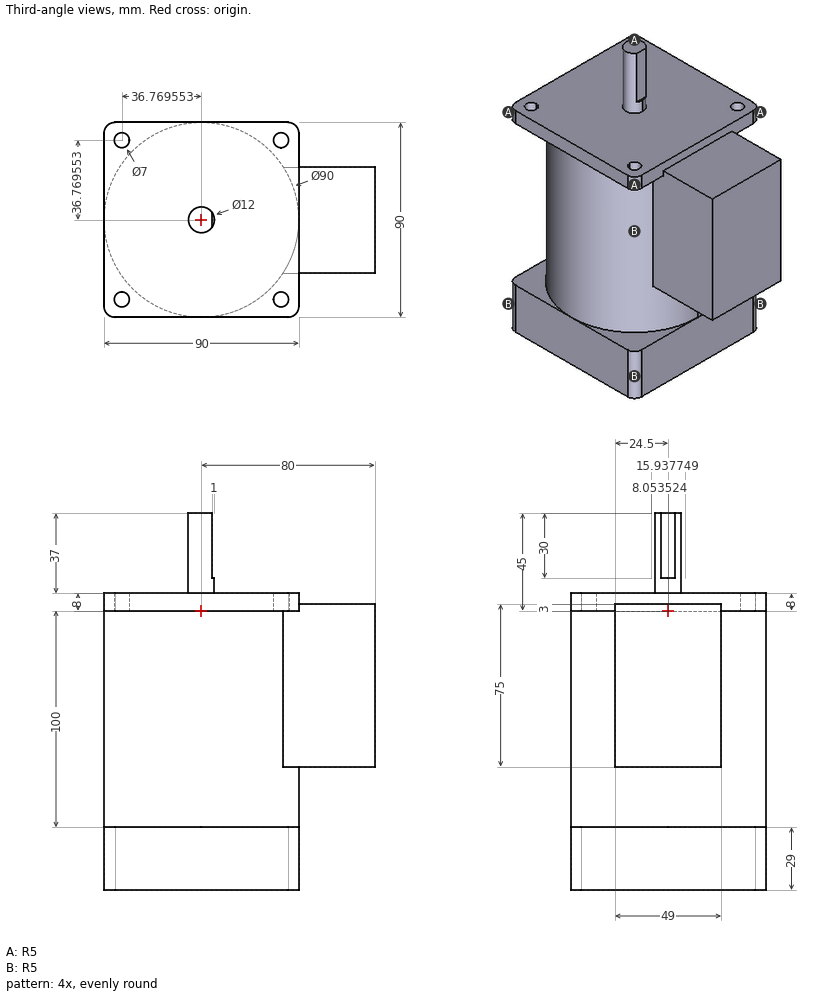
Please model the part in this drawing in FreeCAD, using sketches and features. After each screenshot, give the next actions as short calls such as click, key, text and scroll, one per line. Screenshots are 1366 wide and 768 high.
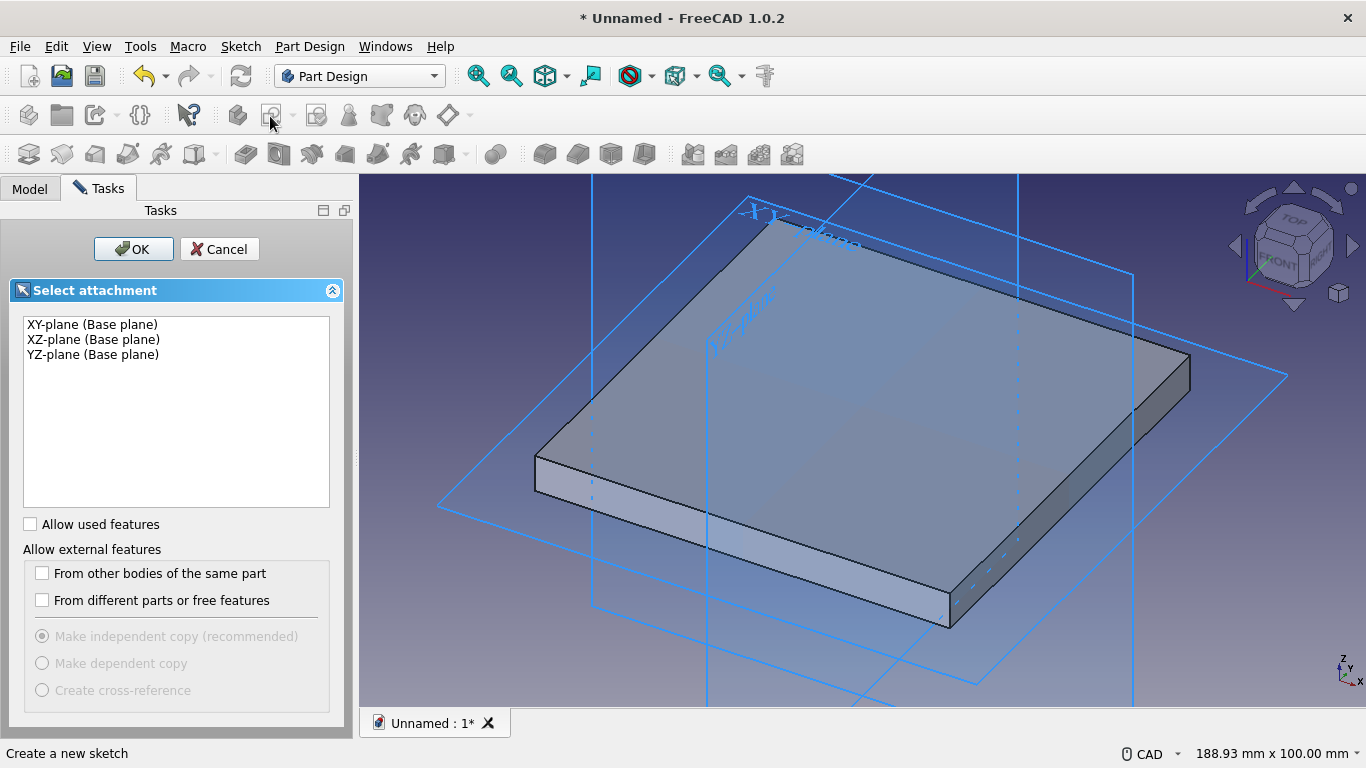
click(84, 324)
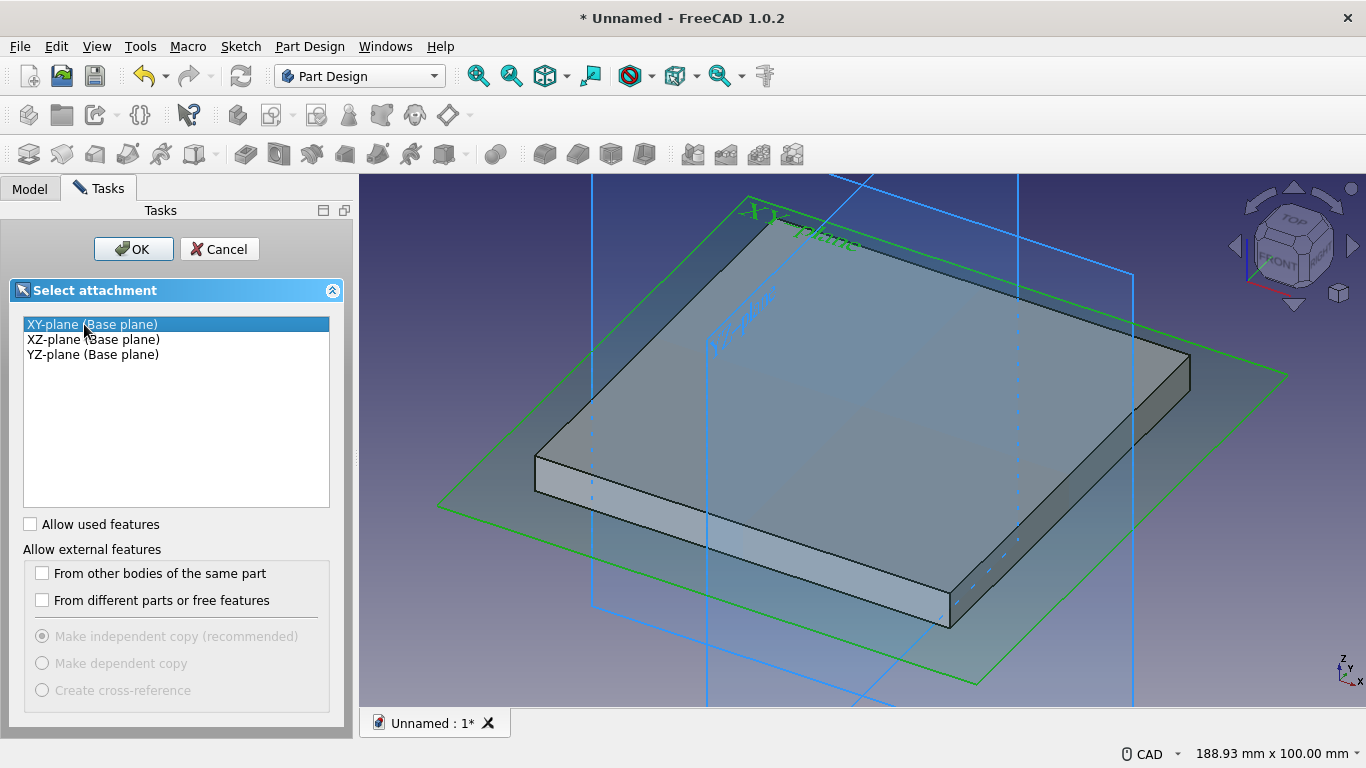
click(134, 249)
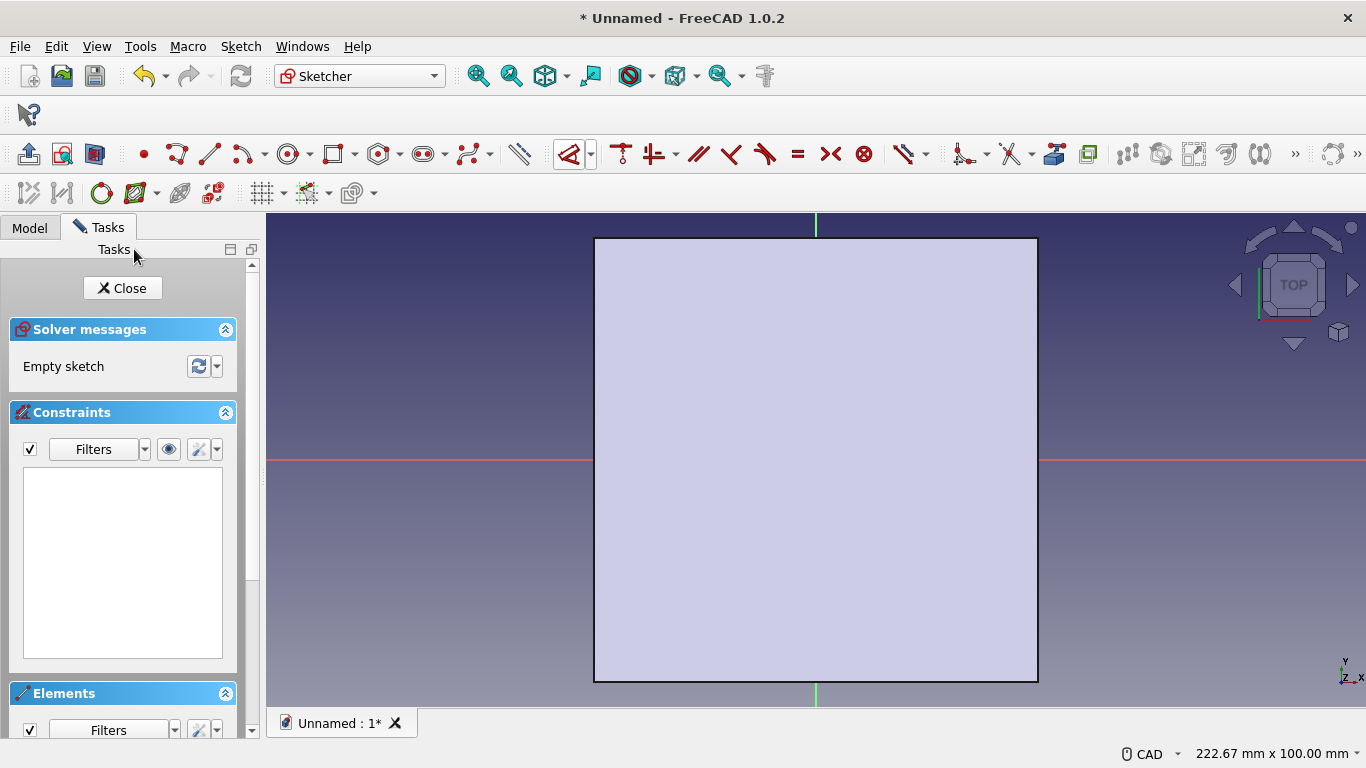
click(95, 154)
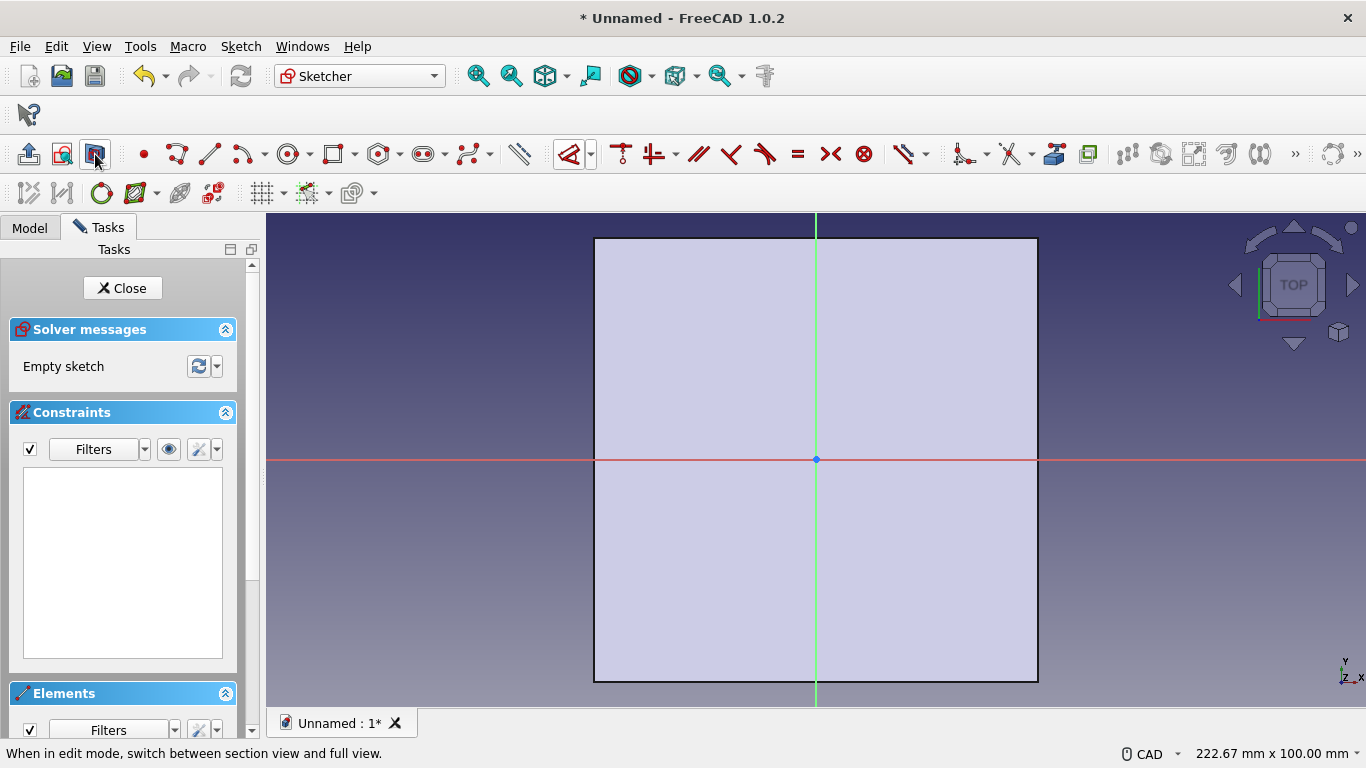
scroll(608, 460, down, 2)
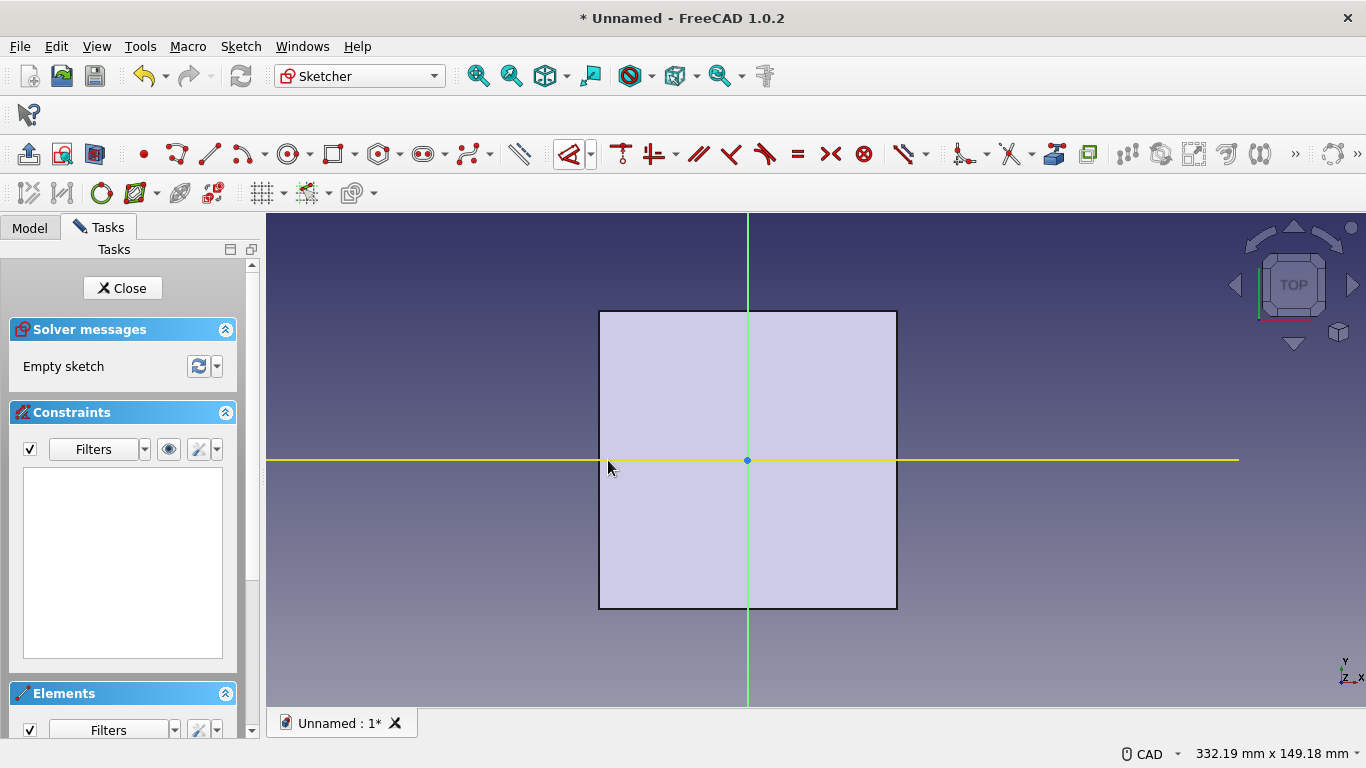
key(g)
key(c)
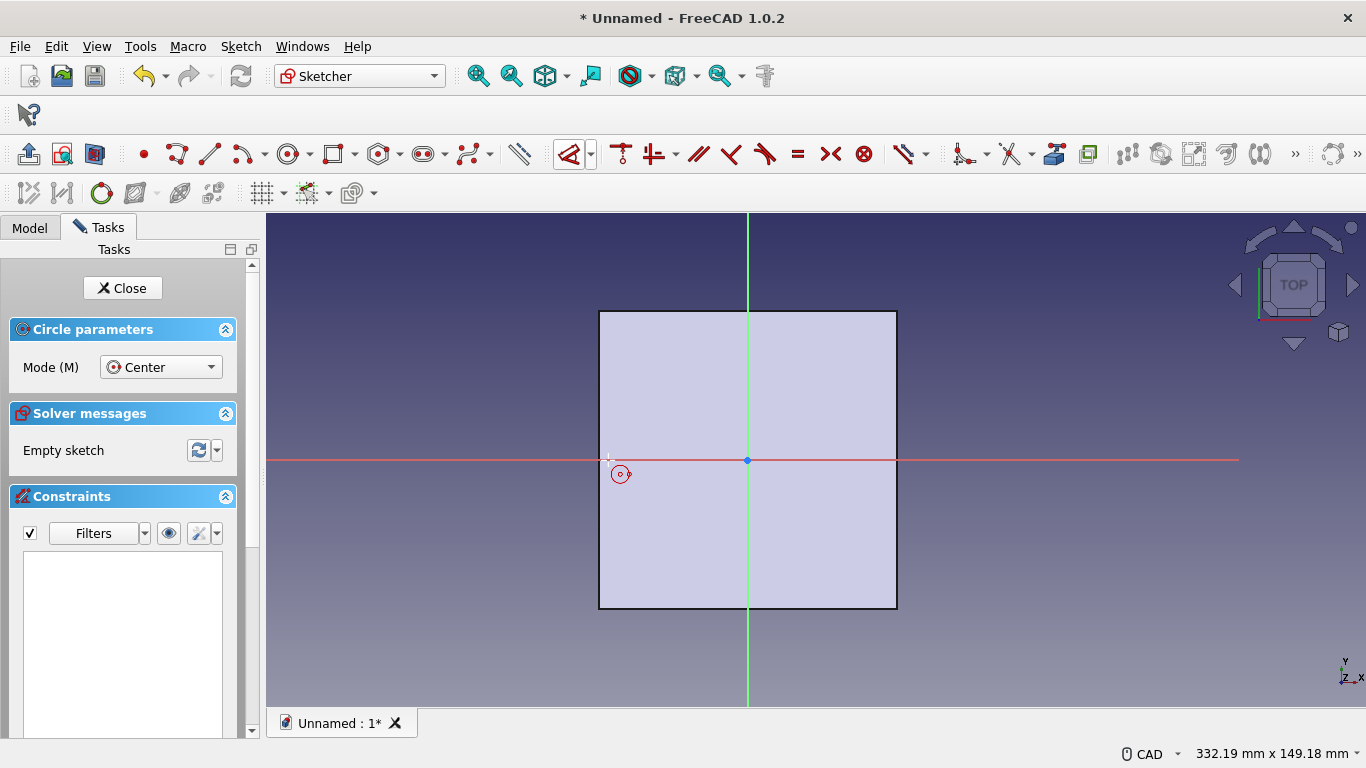
click(748, 460)
click(853, 355)
key(Escape)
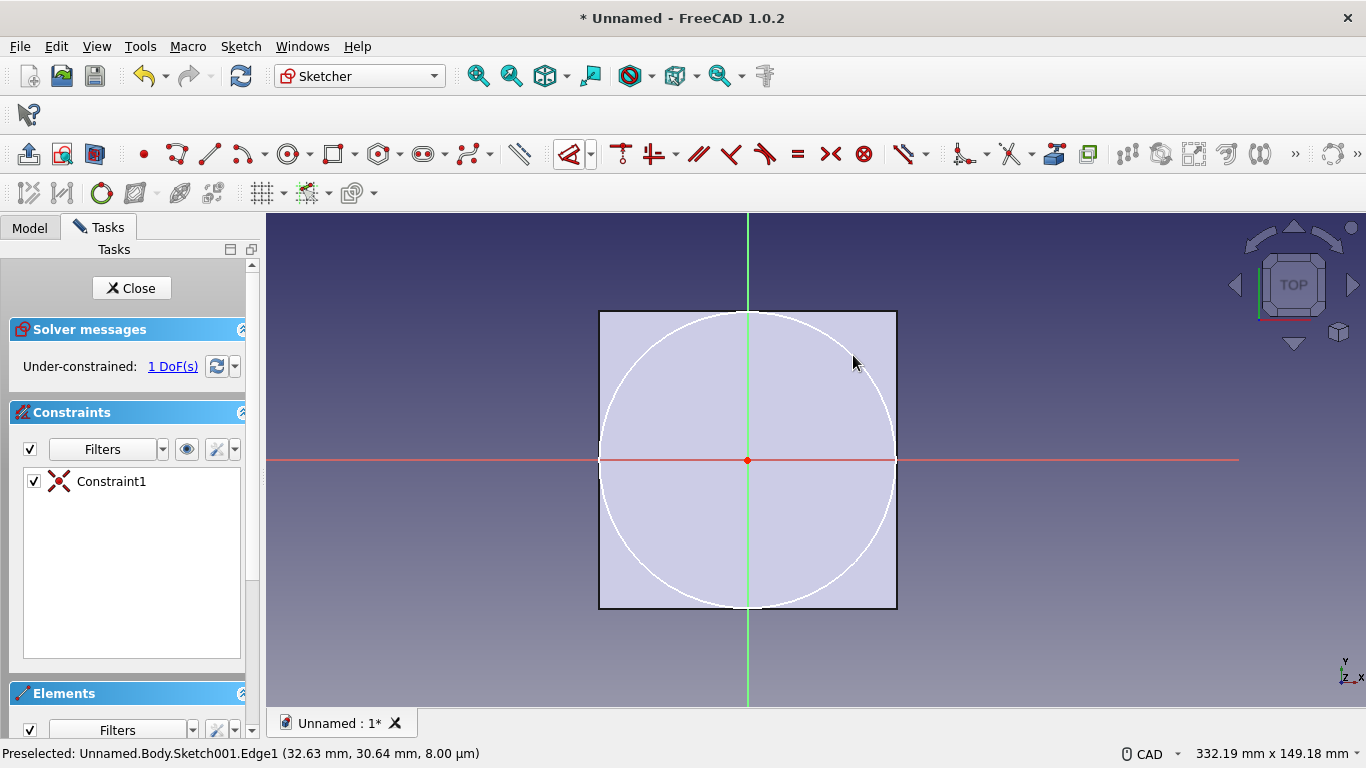
click(852, 355)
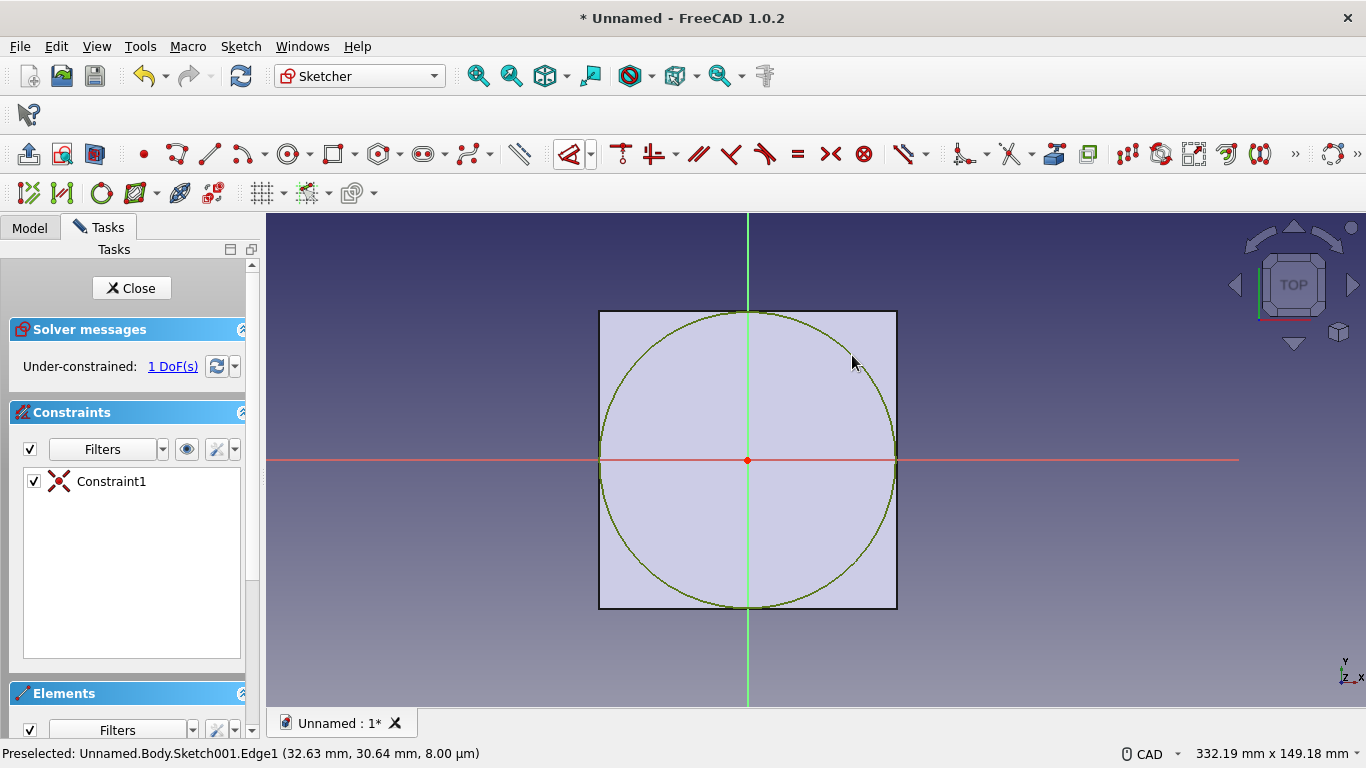
click(590, 154)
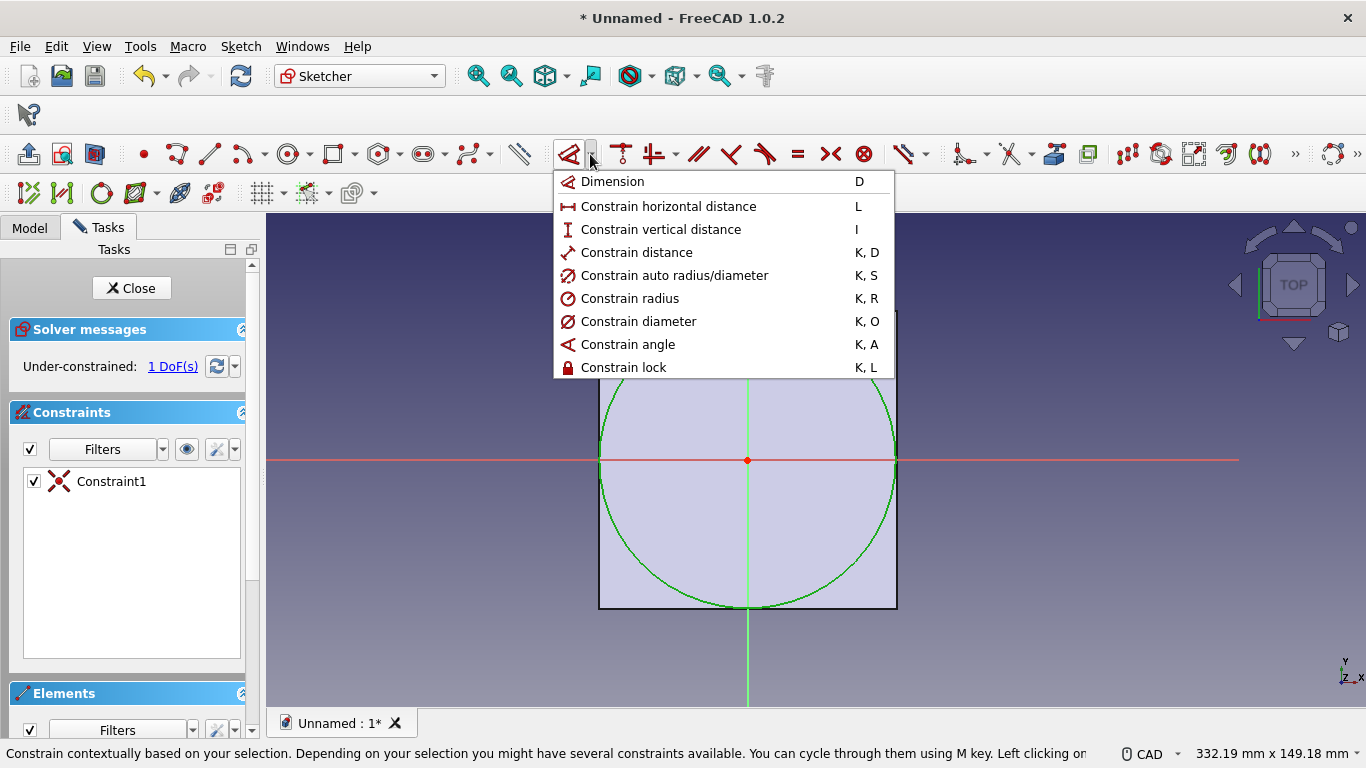
click(724, 322)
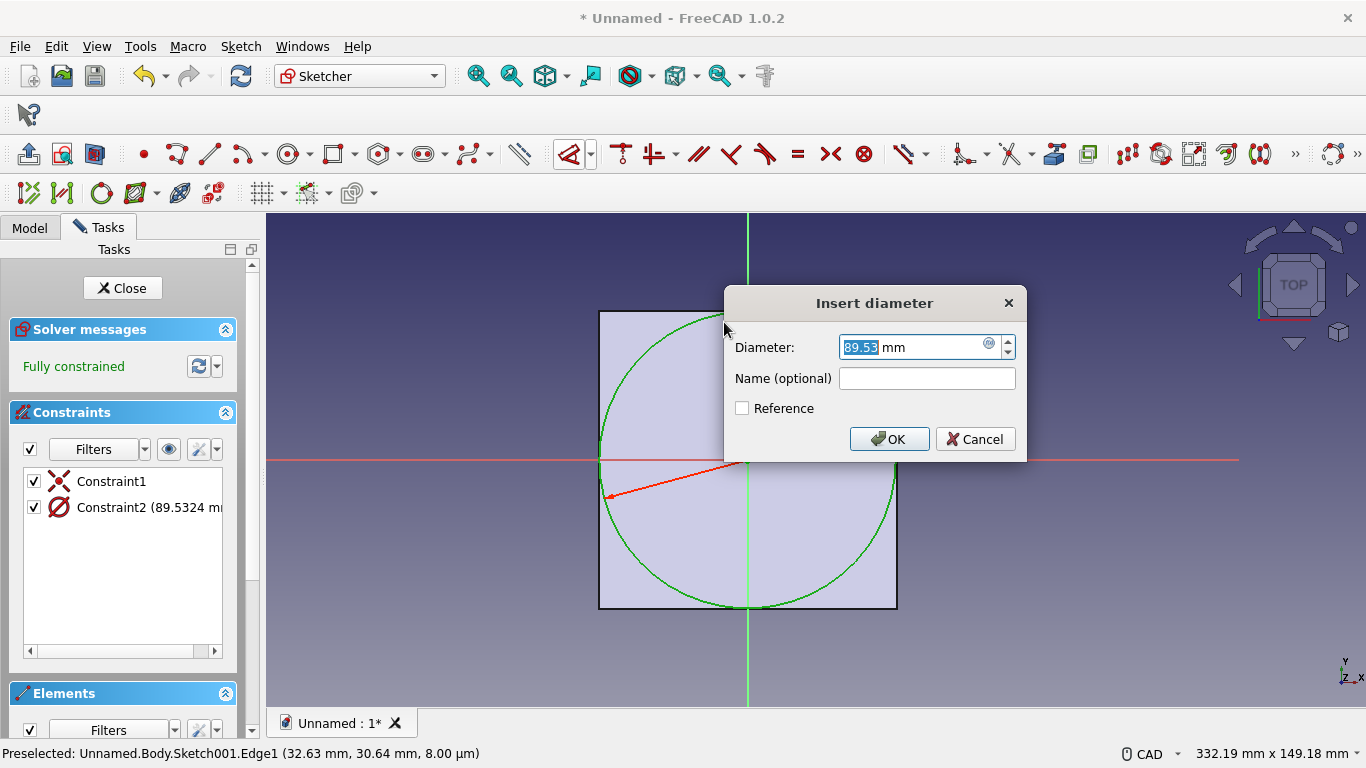
text(90)
key(Return)